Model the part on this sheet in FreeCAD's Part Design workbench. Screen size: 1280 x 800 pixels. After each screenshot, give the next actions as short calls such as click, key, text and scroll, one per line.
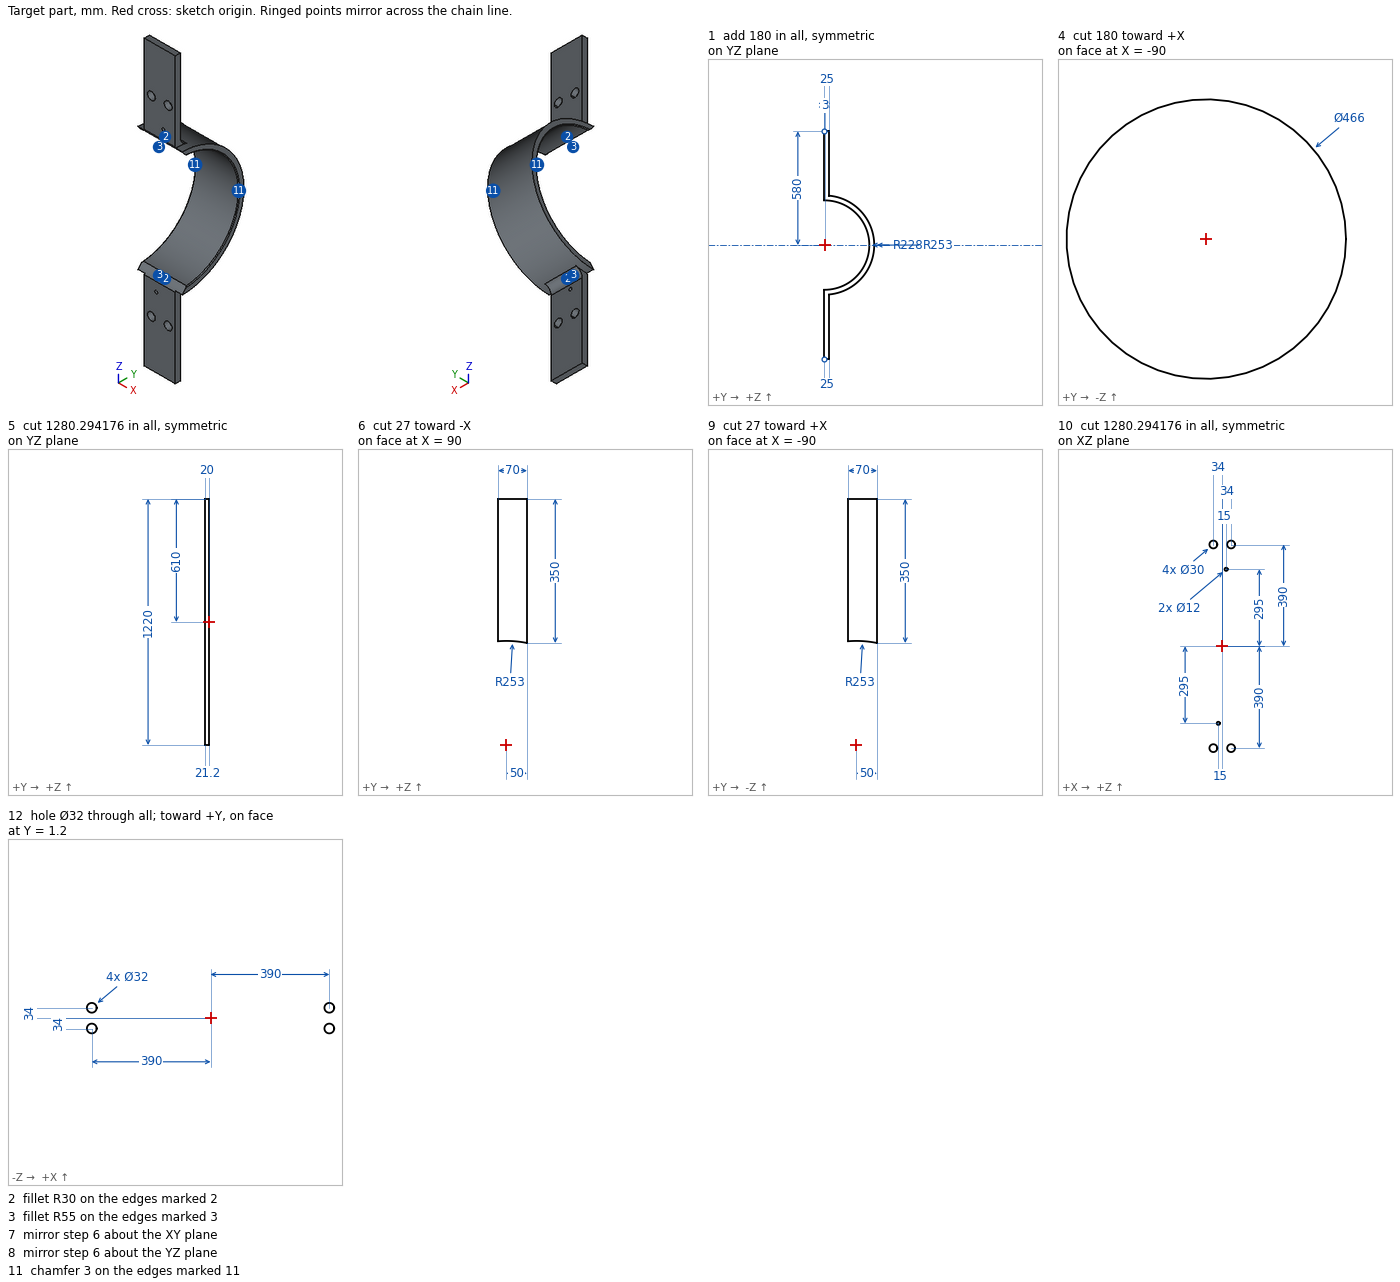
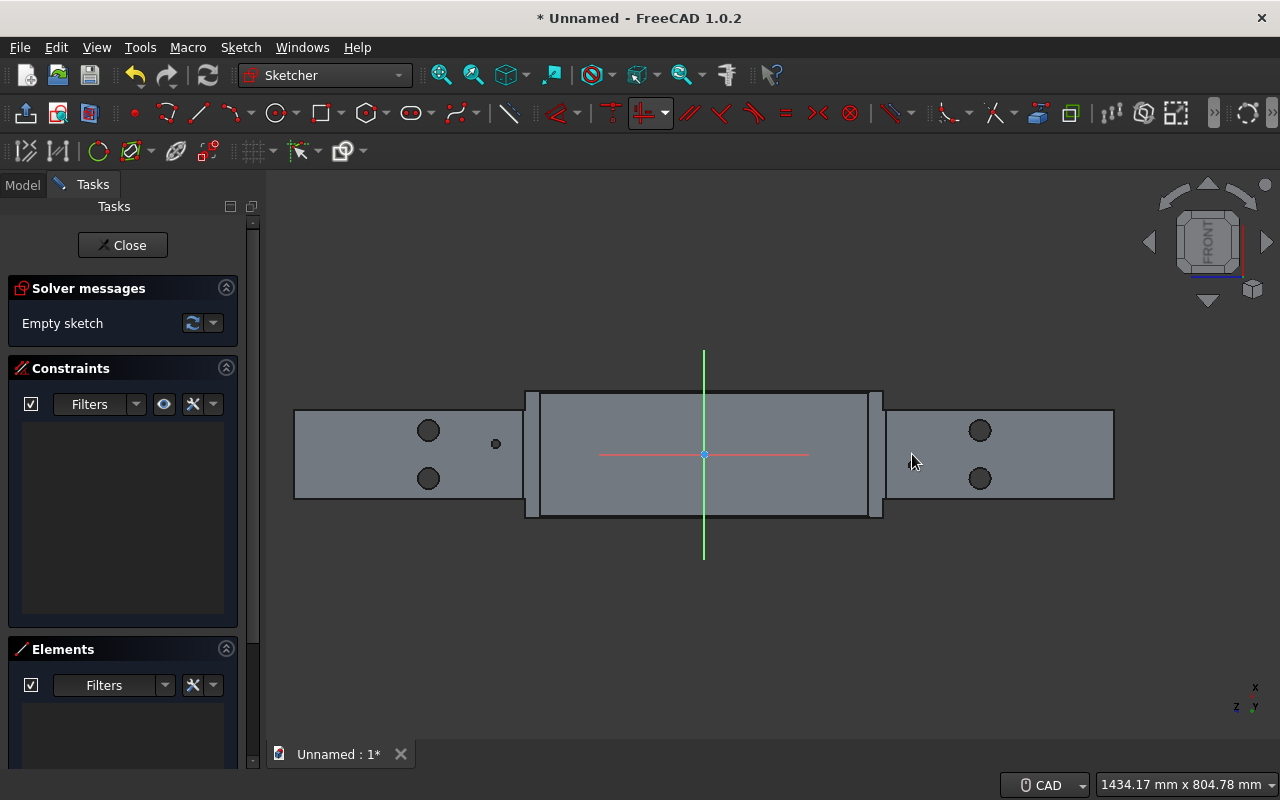
click(276, 114)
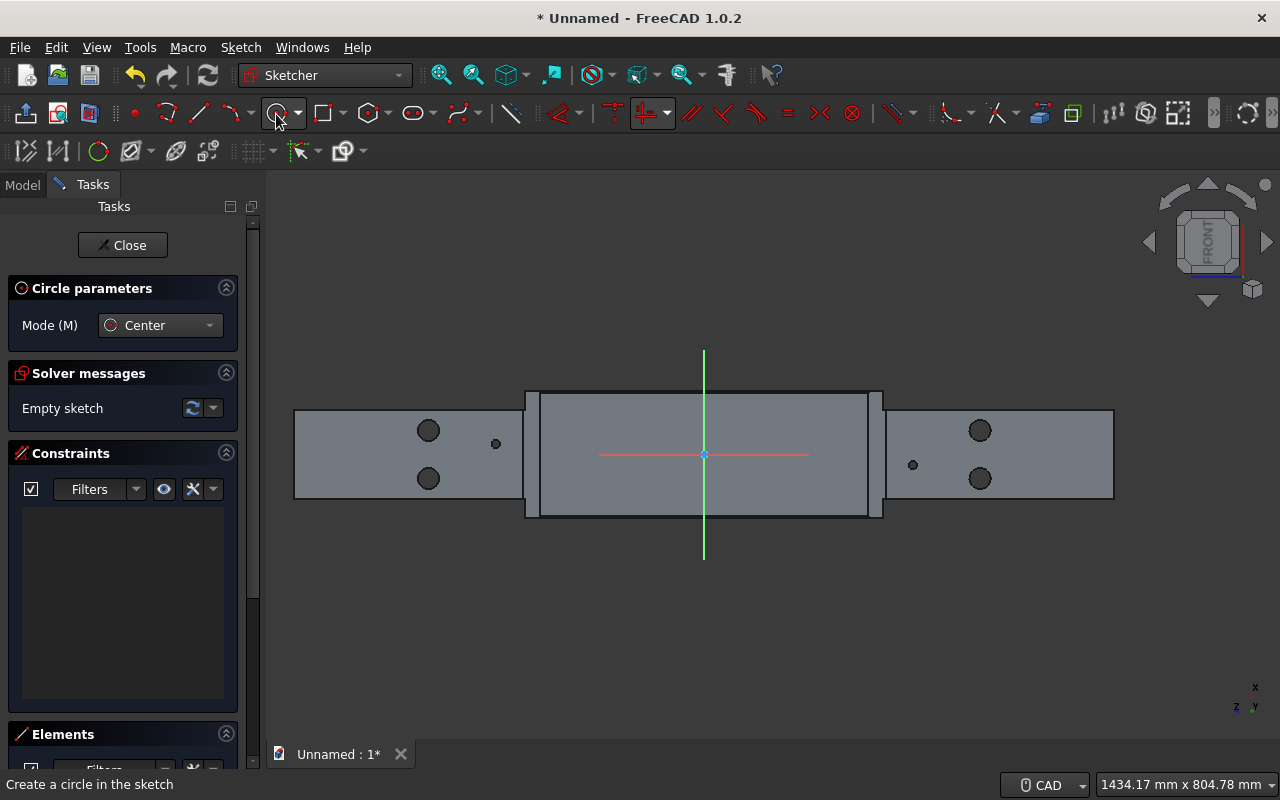
scroll(429, 479, up, 4)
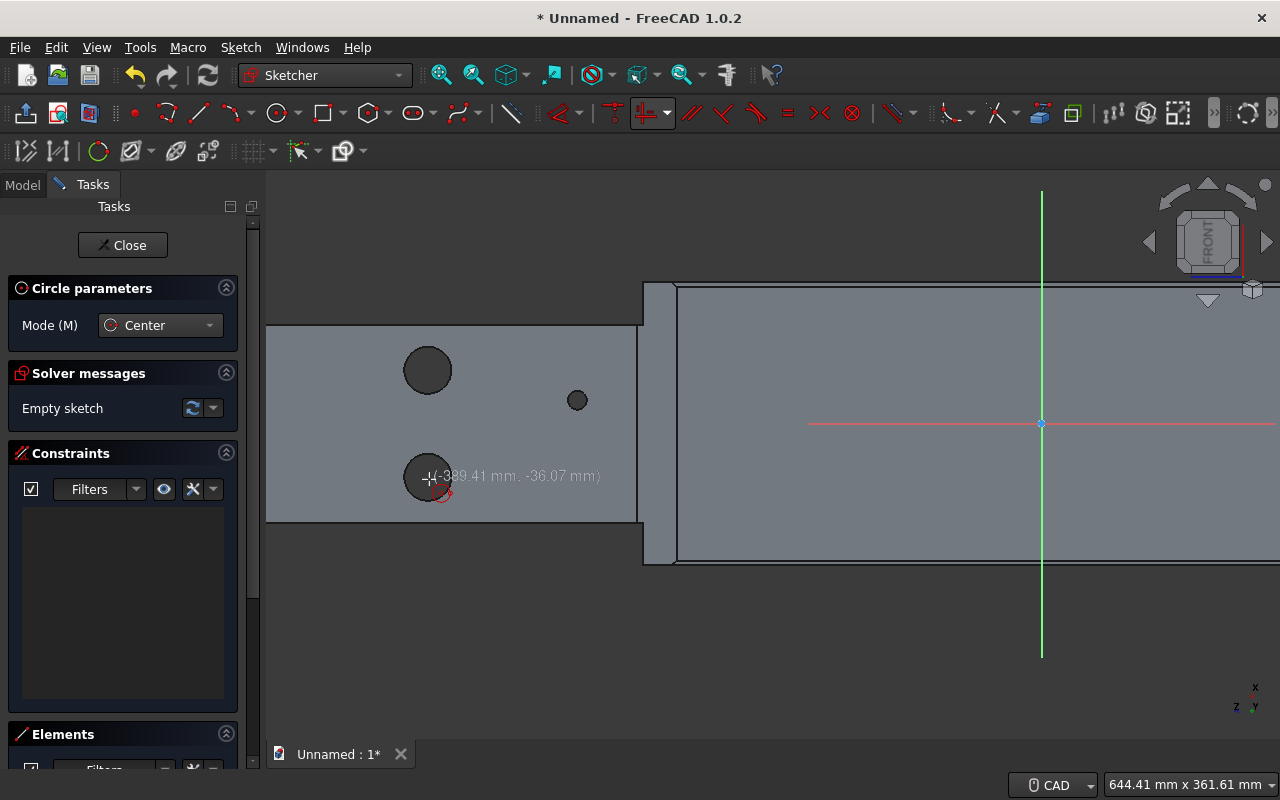
click(428, 477)
move(446, 460)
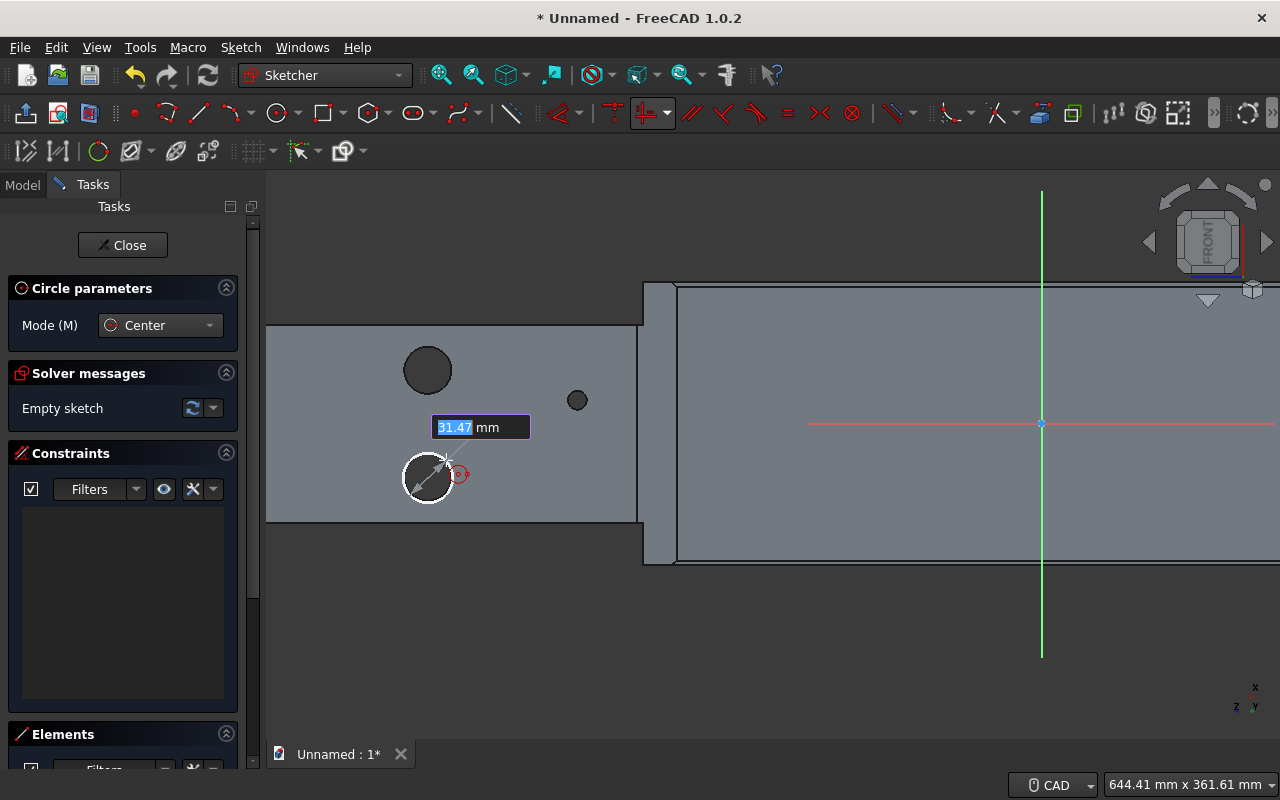
text(32)
key(Return)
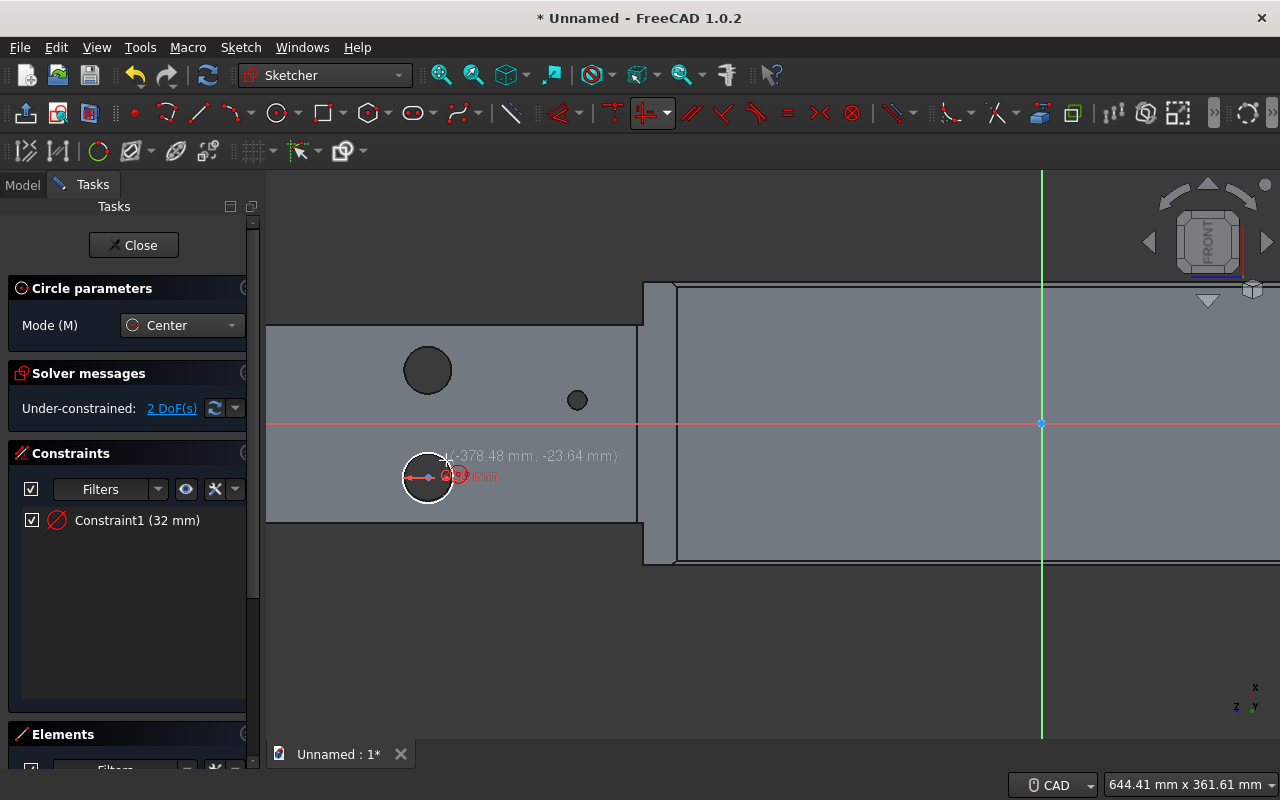
click(428, 370)
move(446, 353)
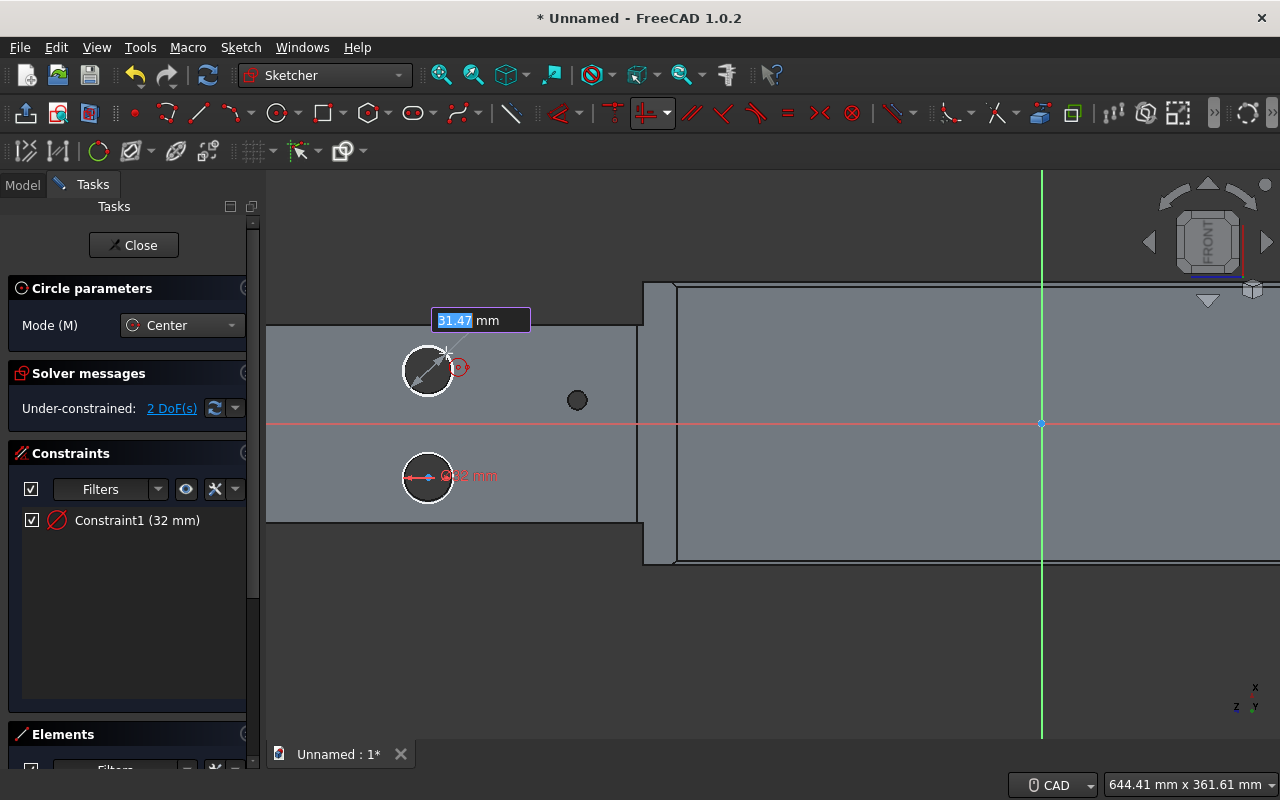
text(32)
key(Return)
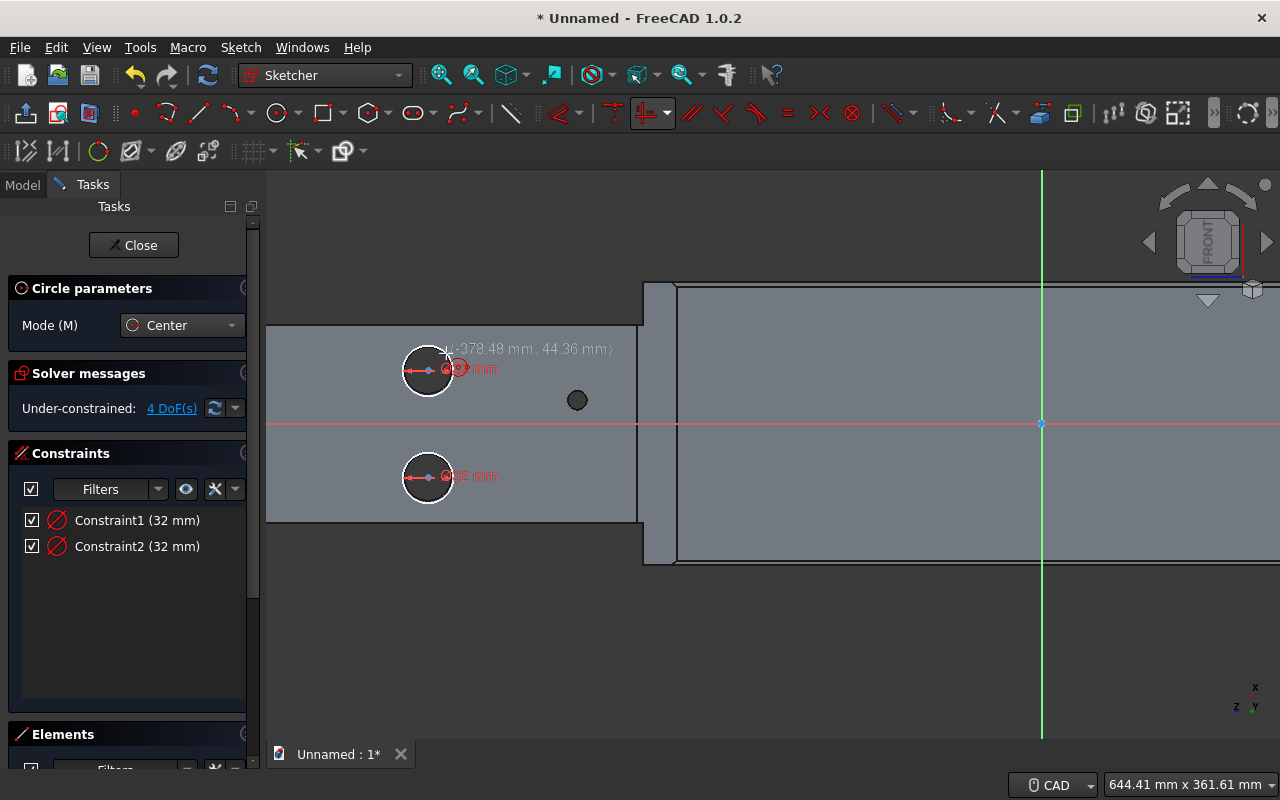
scroll(429, 480, down, 4)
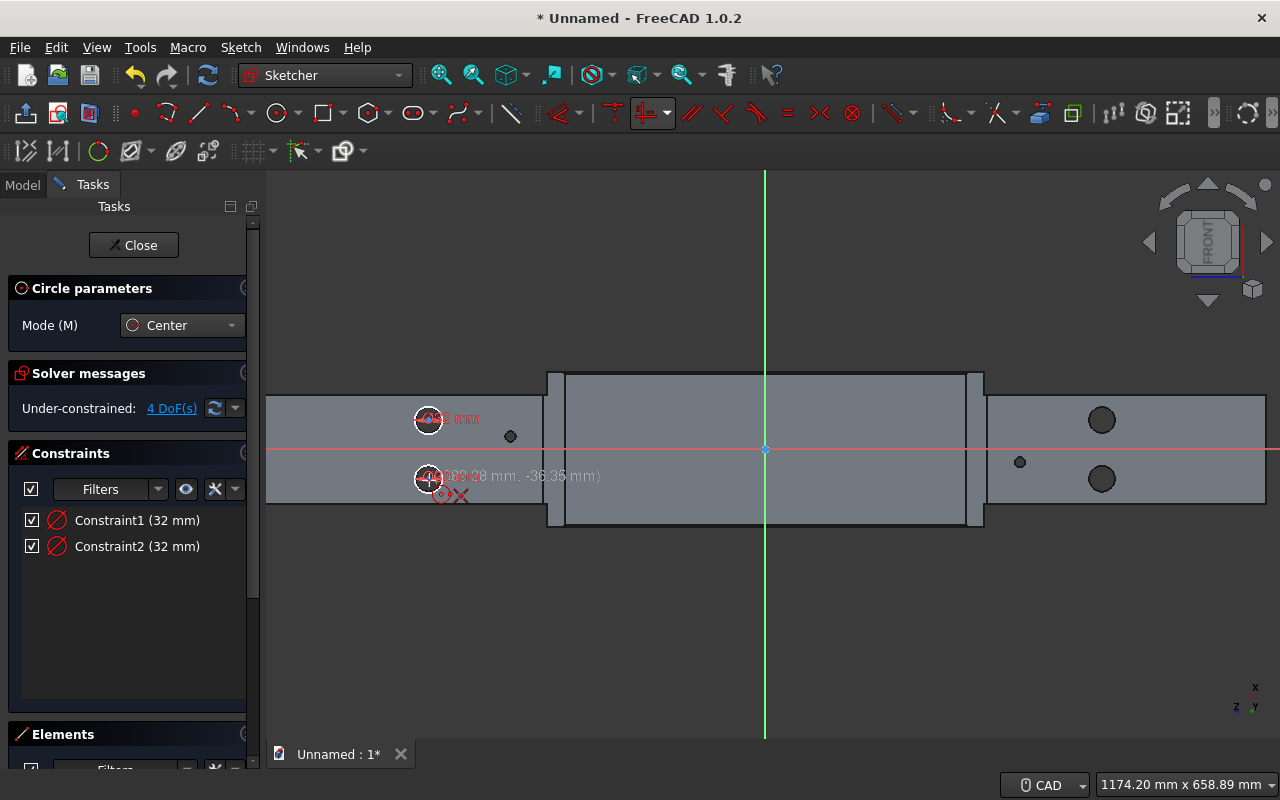
scroll(980, 431, up, 4)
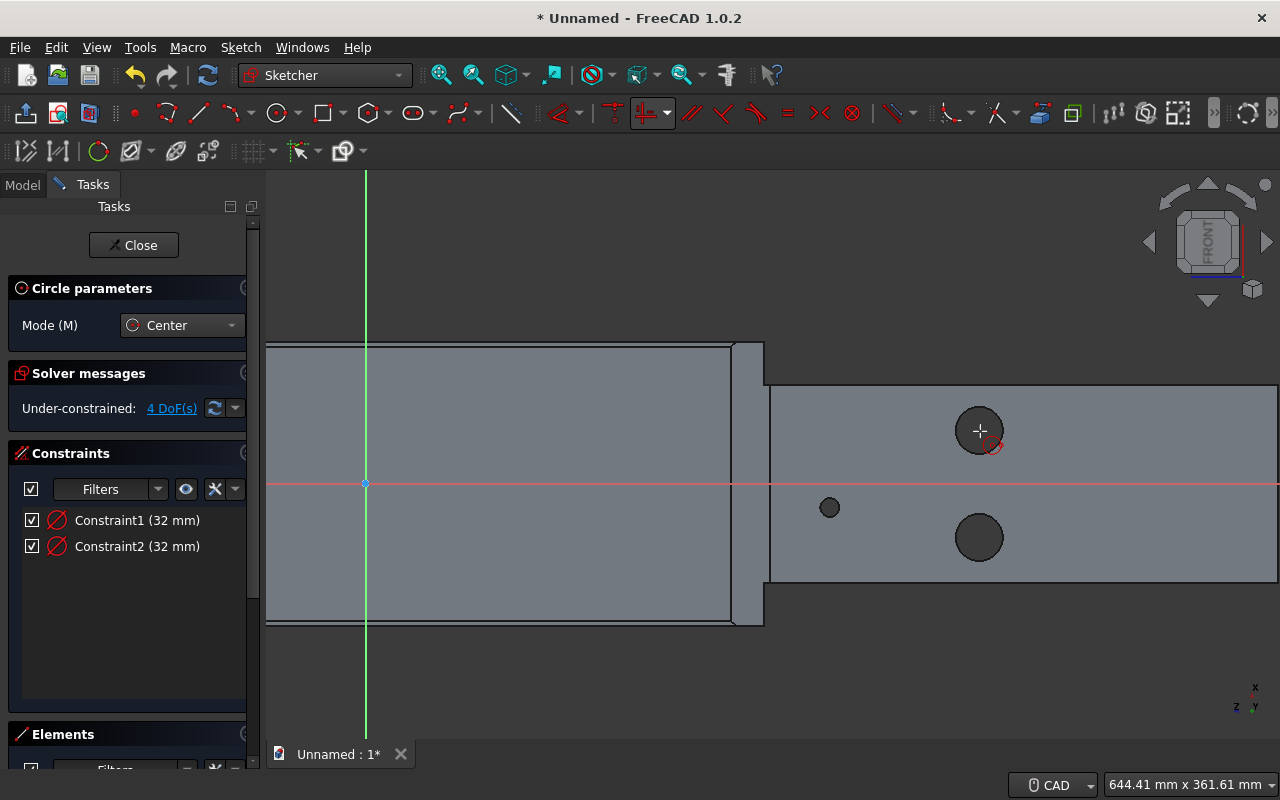
click(979, 430)
move(997, 413)